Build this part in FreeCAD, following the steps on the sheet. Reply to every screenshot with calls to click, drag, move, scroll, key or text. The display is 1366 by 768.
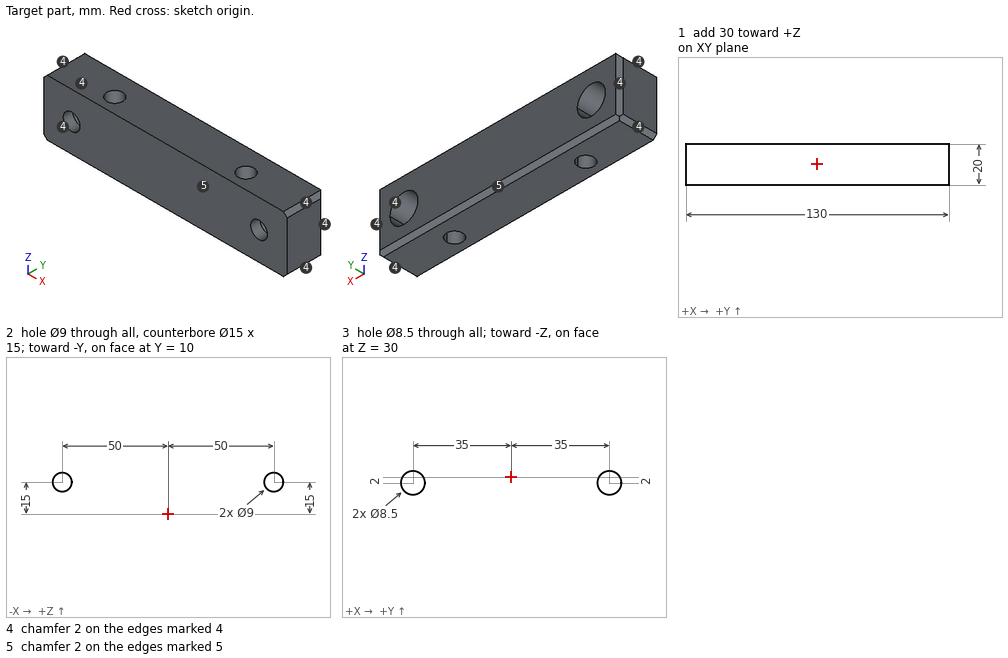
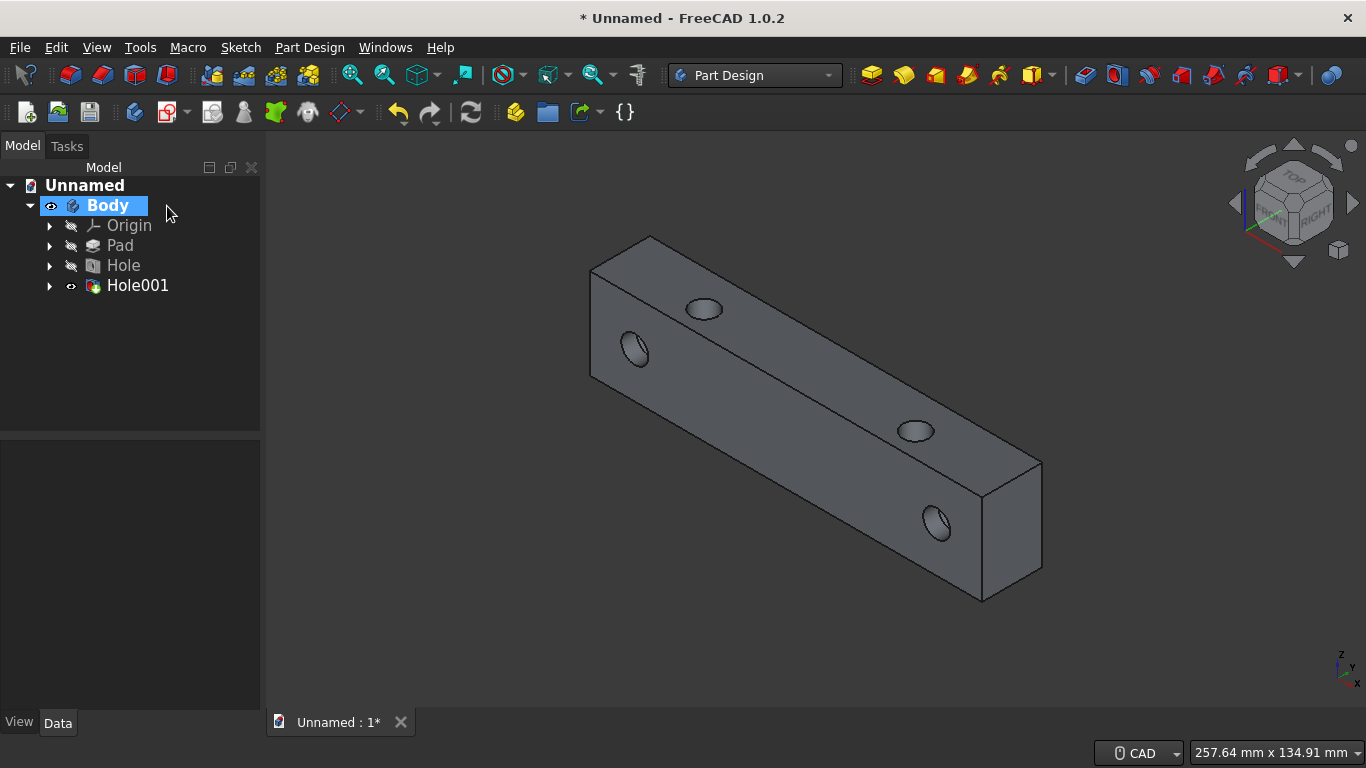
click(1012, 479)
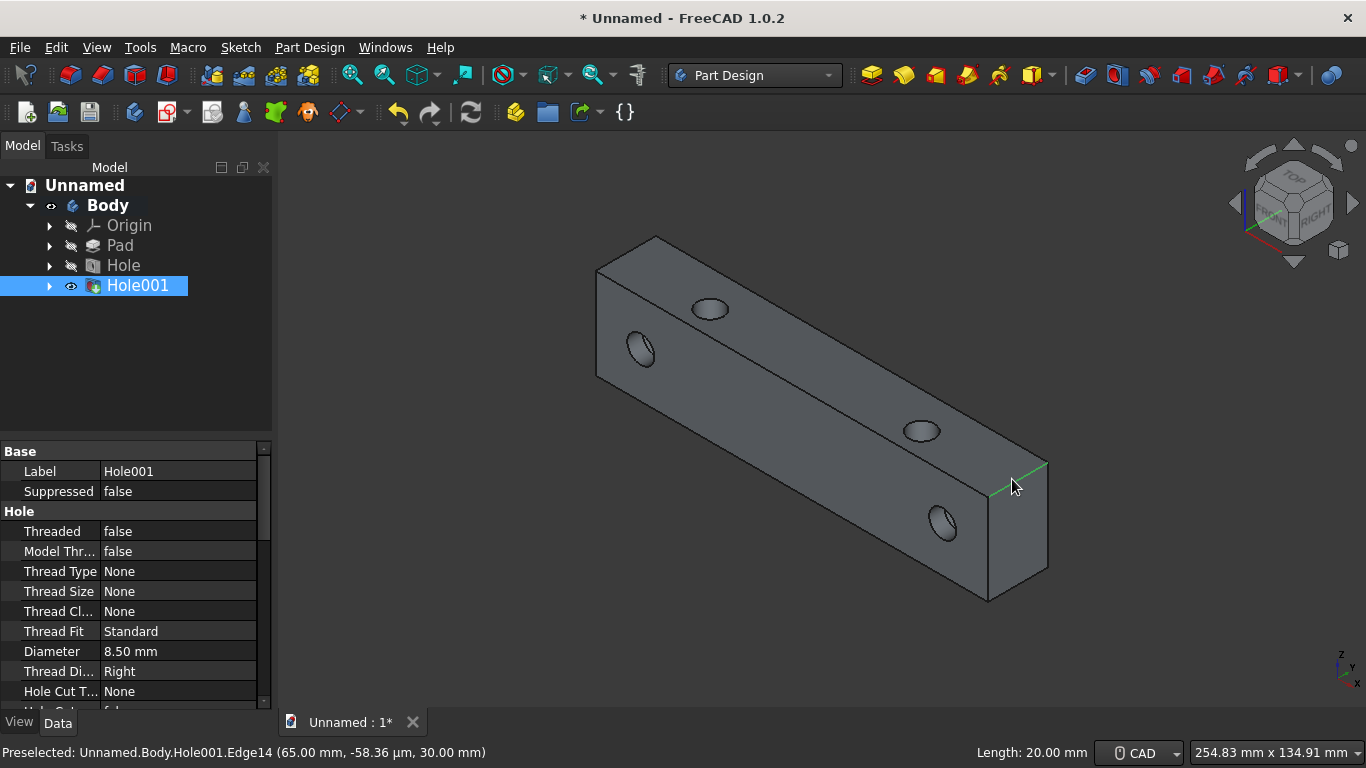
key(2)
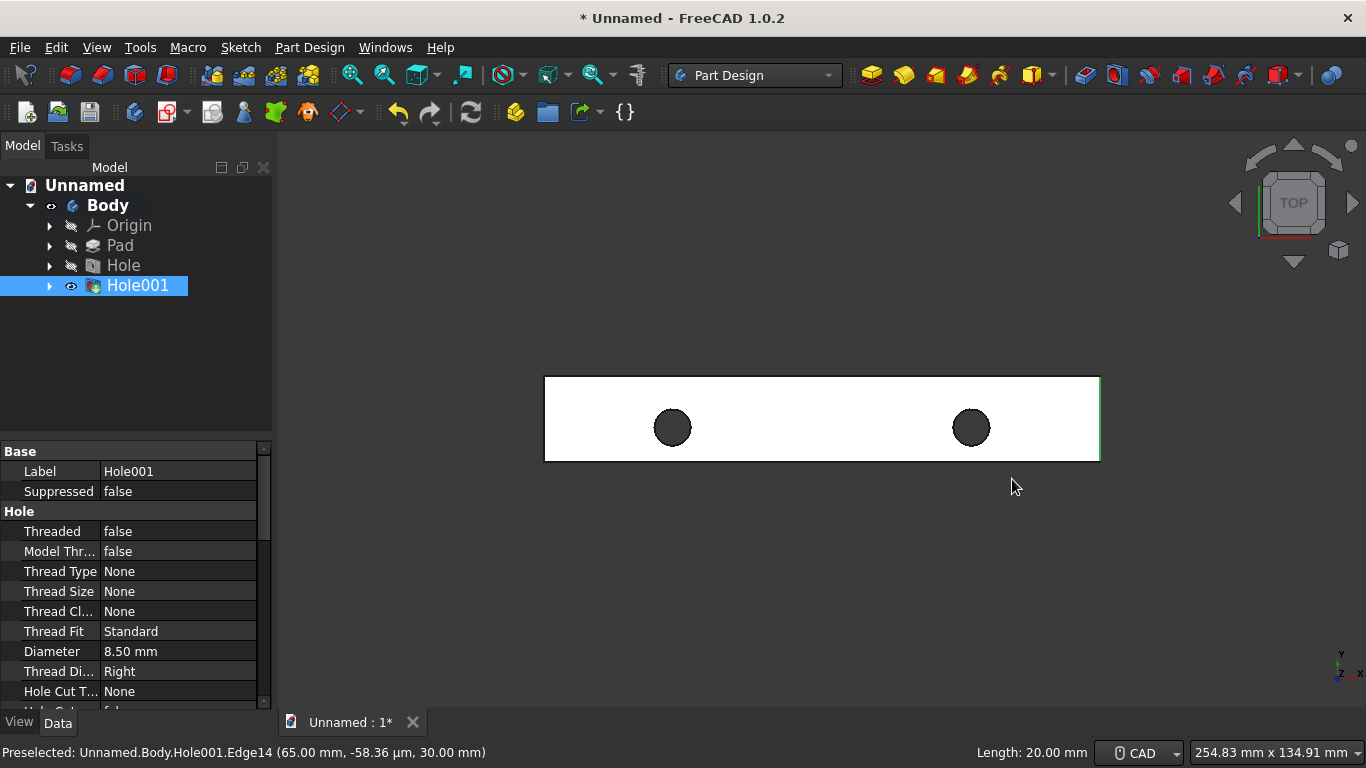
click(544, 418, ctrl)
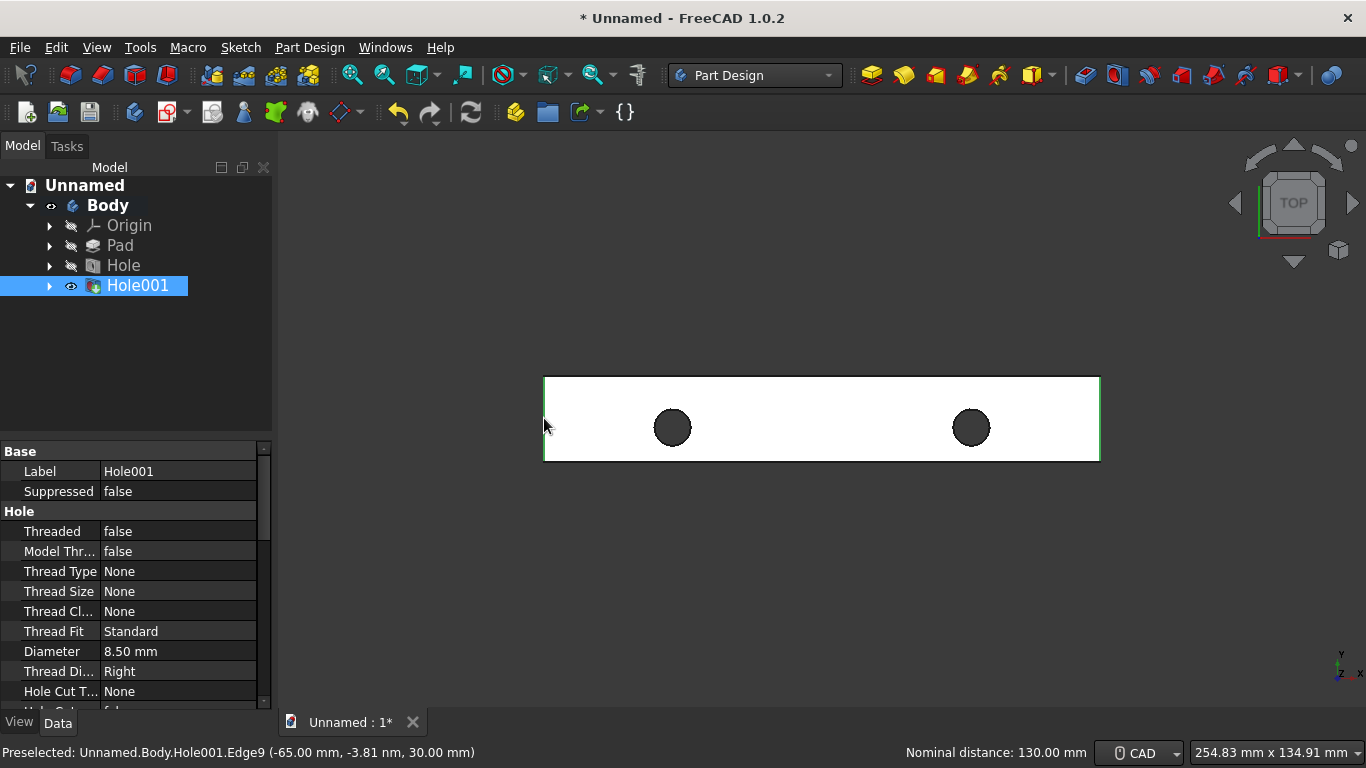
key(0)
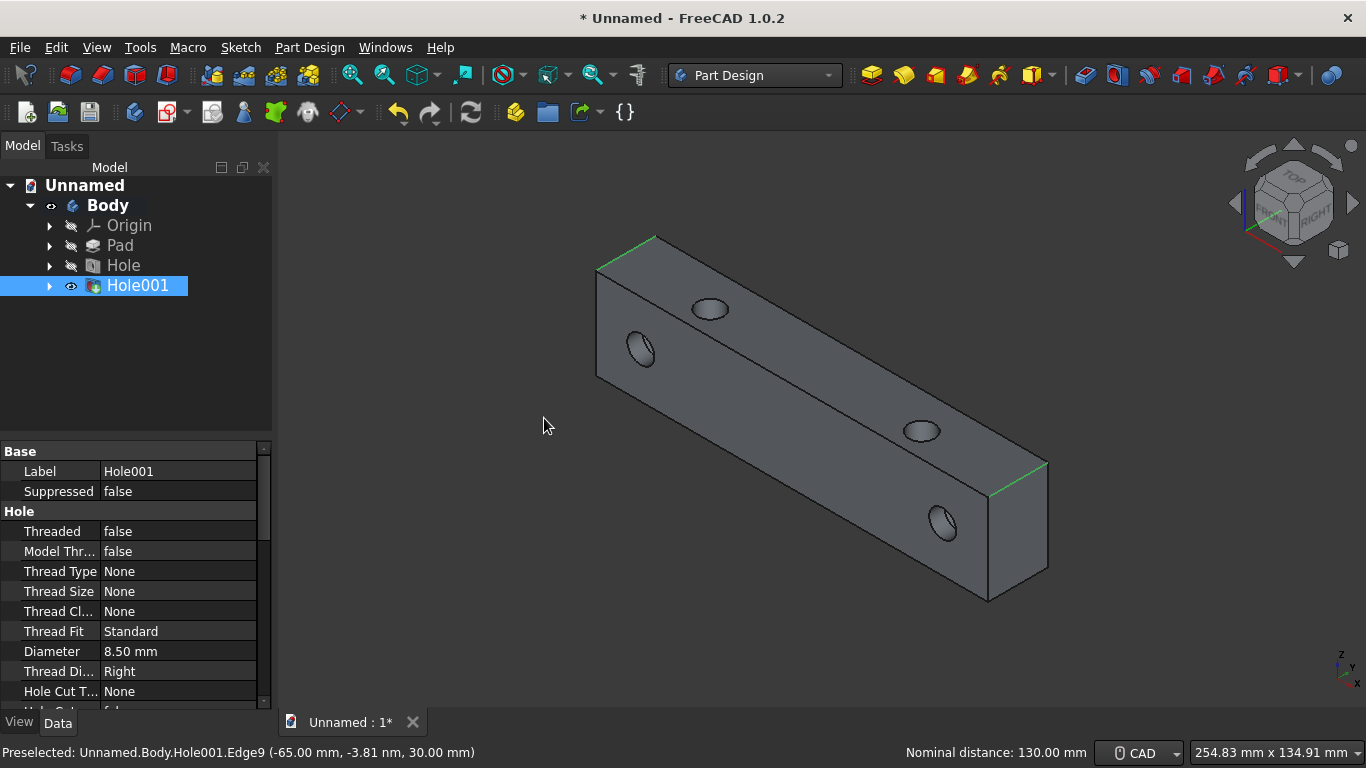
key(1)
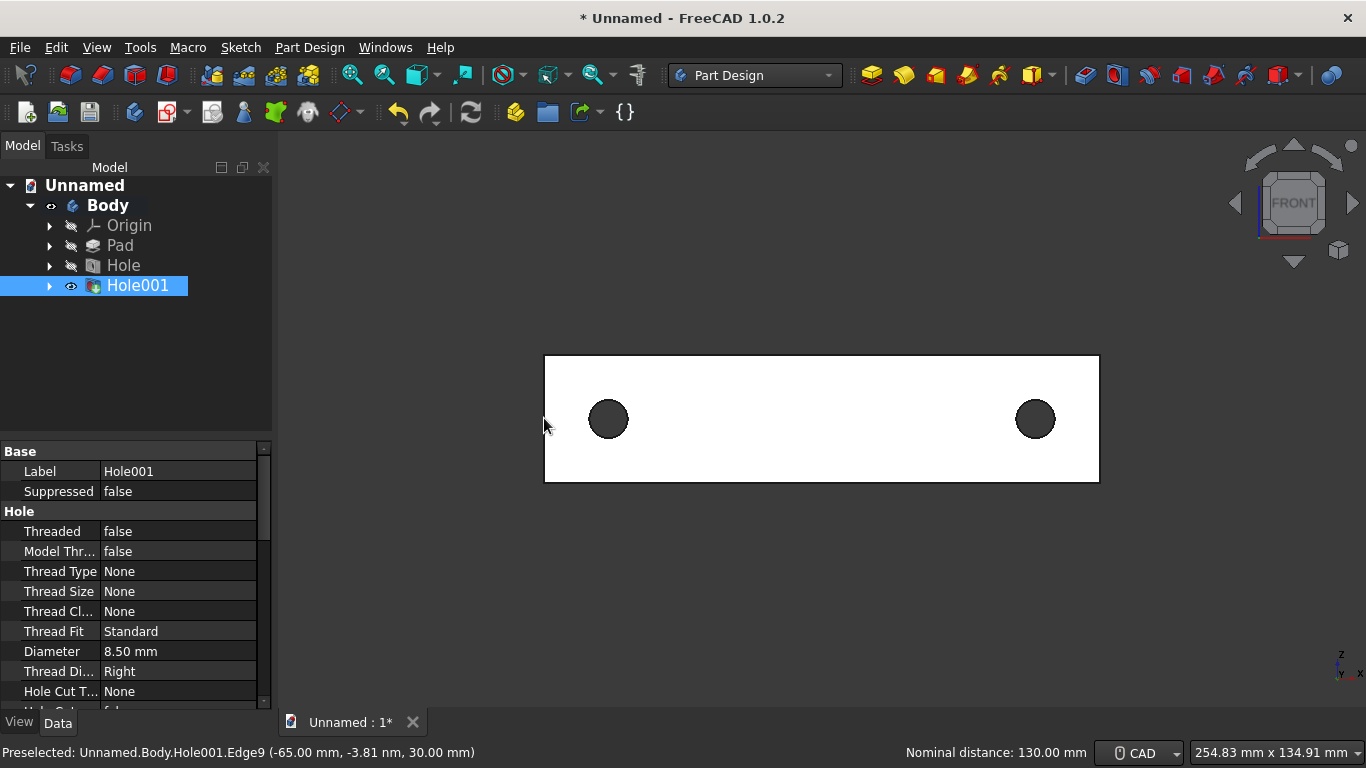
key(3)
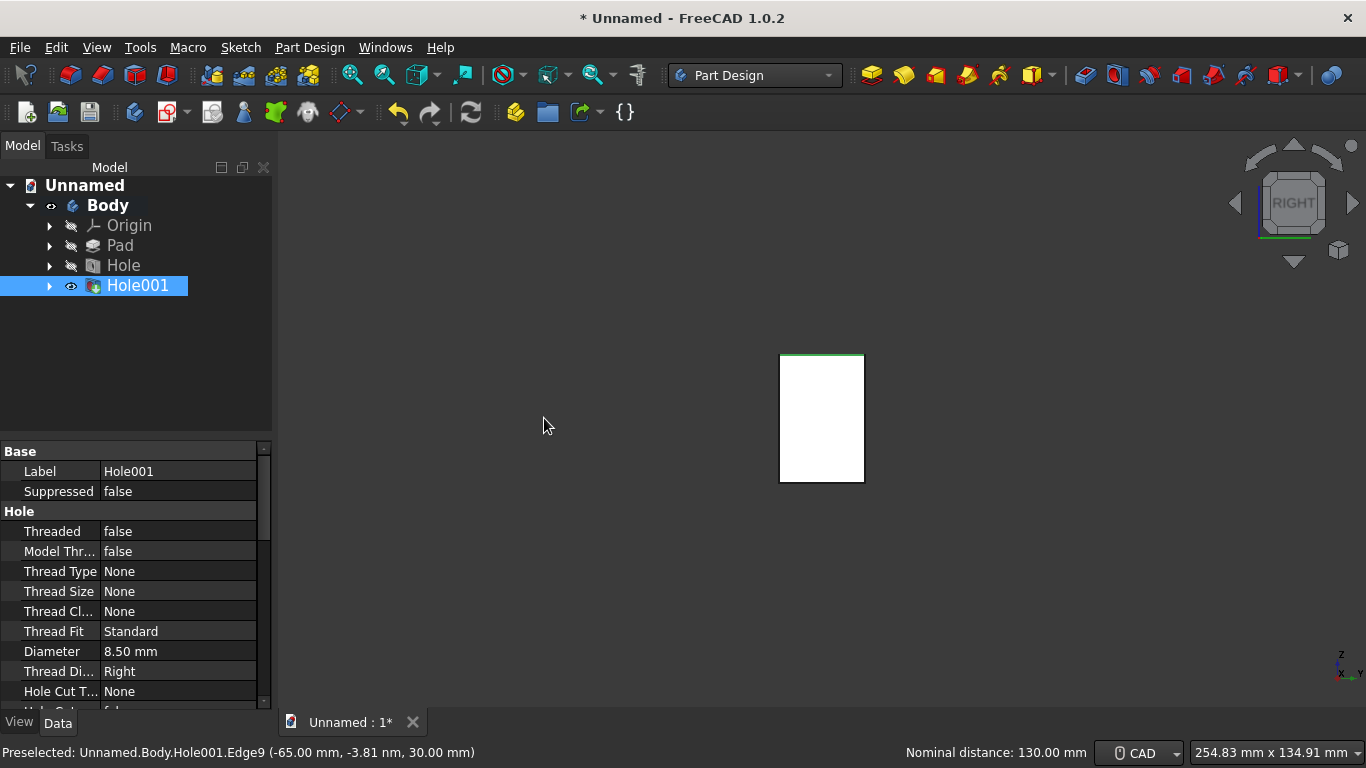
key(v)
key(f)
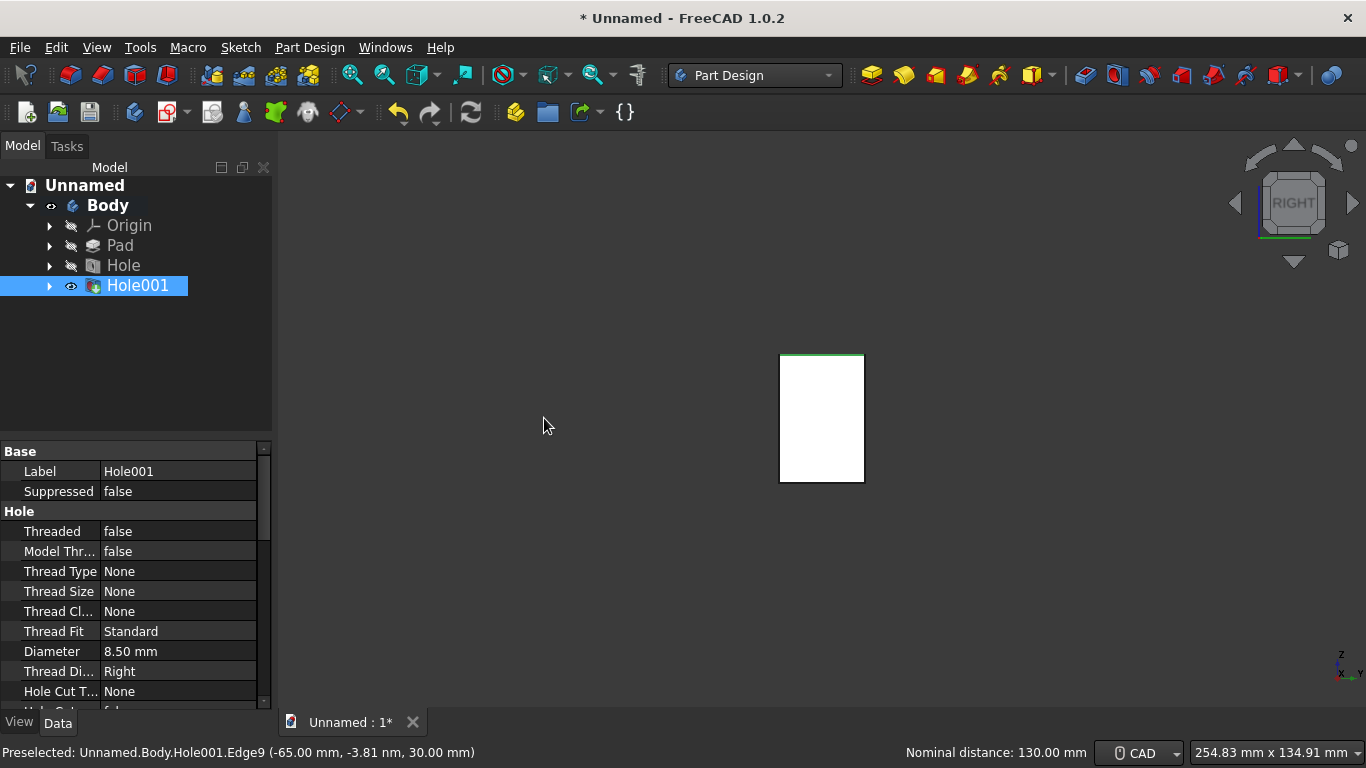
click(822, 482, ctrl)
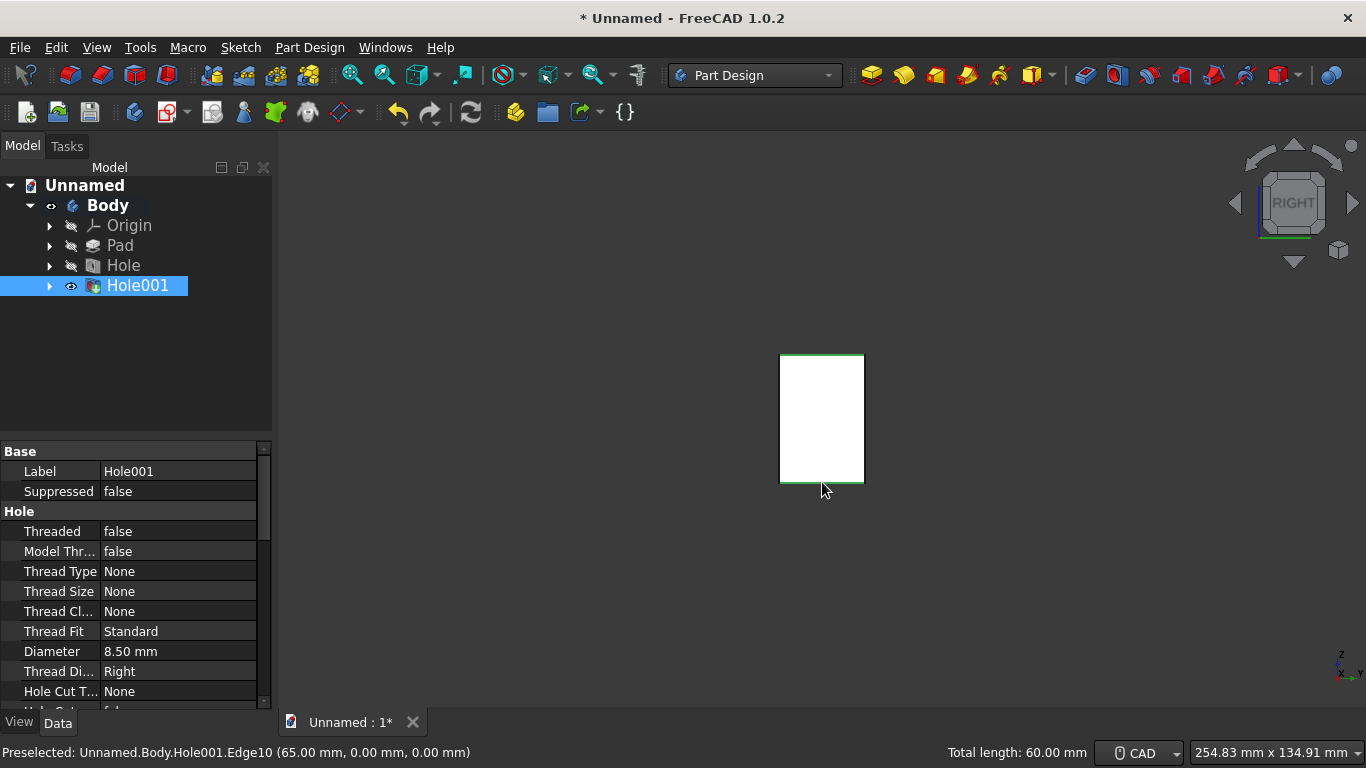
click(865, 418, ctrl)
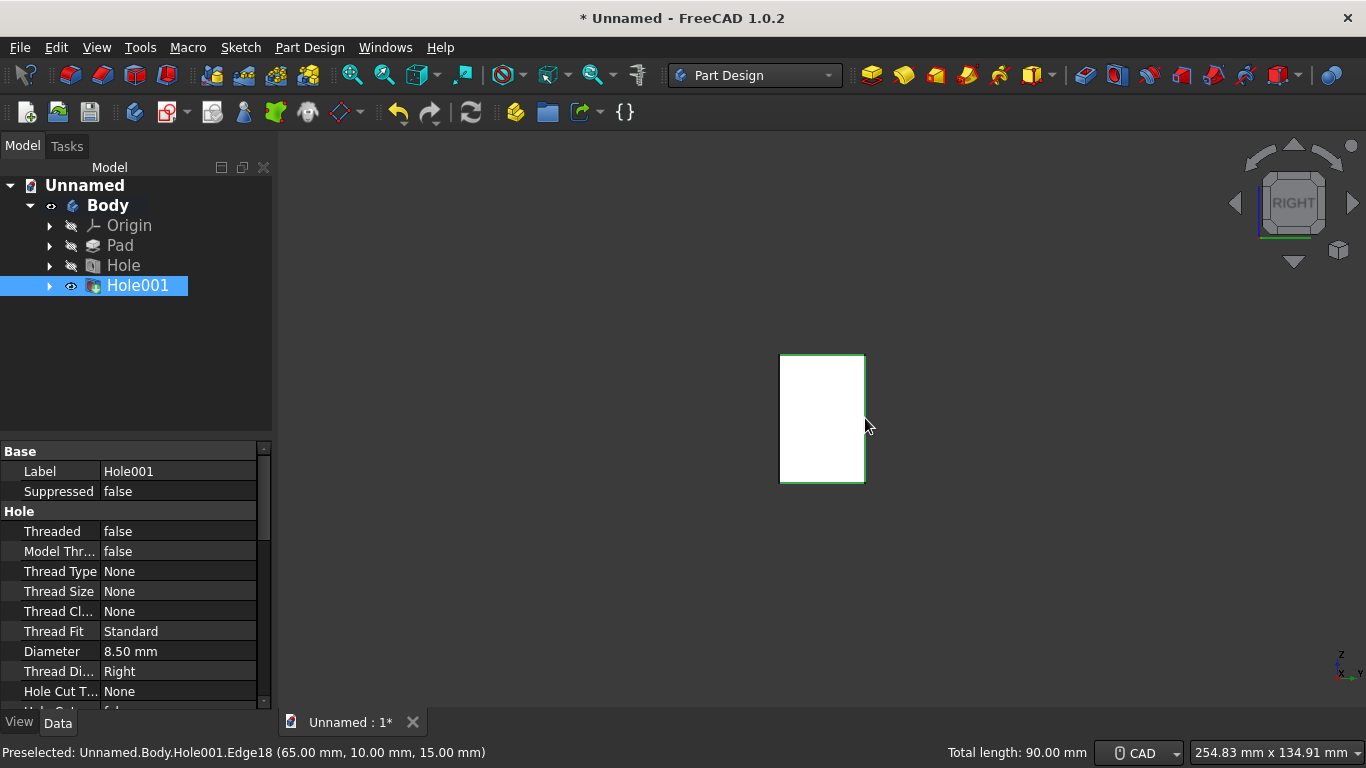
key(5)